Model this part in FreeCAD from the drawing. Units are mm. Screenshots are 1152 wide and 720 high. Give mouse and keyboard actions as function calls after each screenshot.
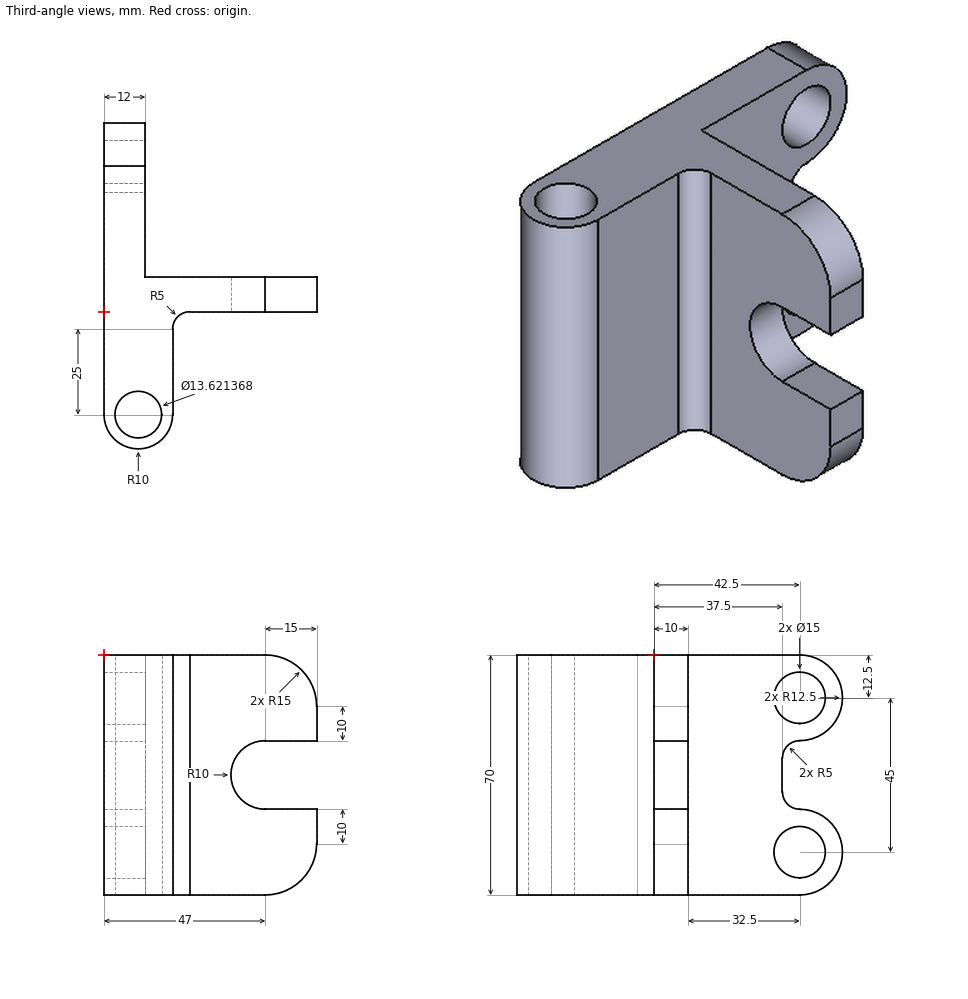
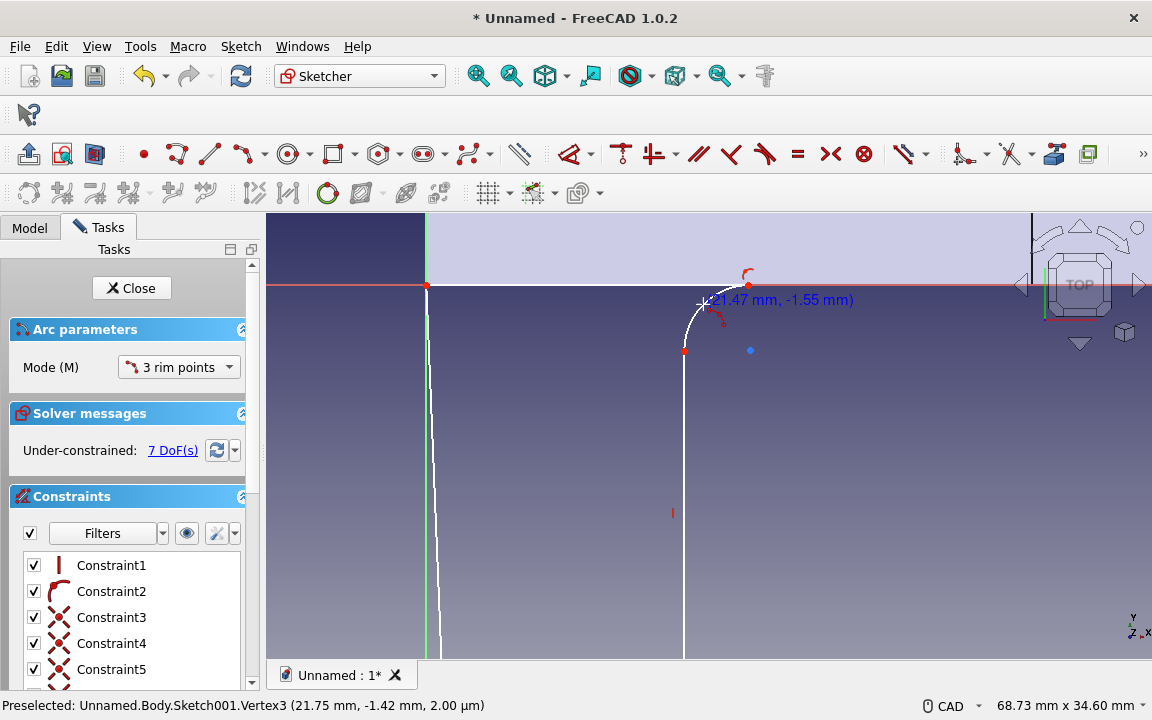
scroll(705, 306, down, 3)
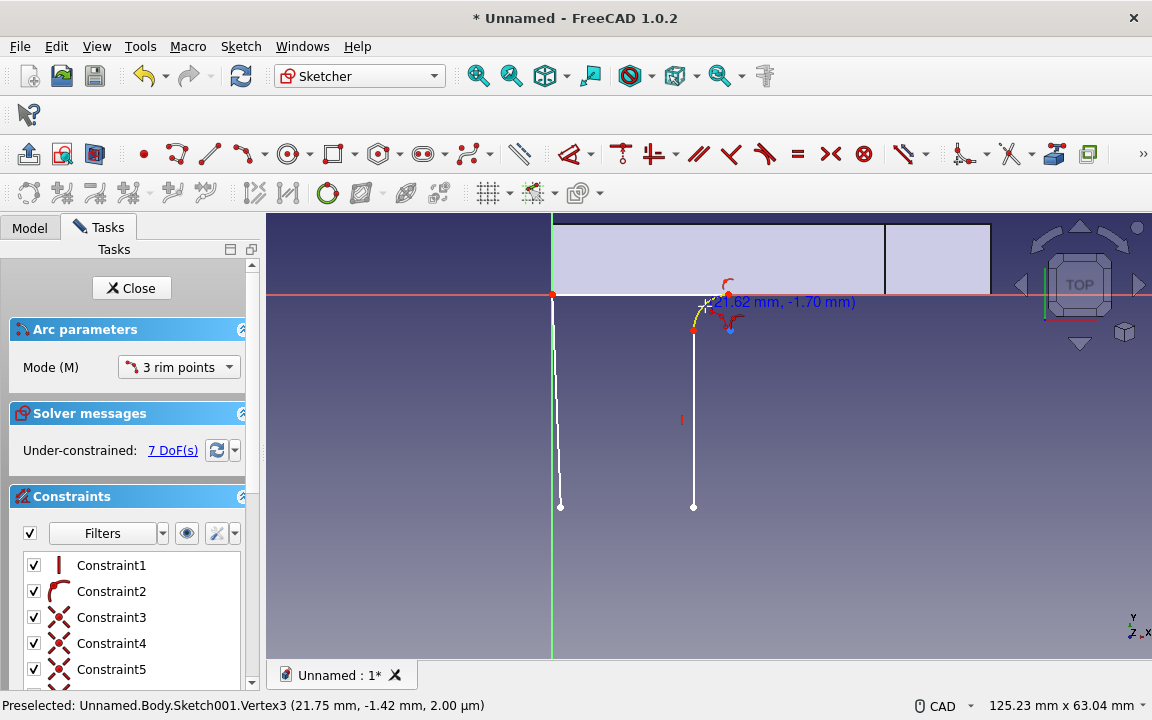
click(561, 508)
click(694, 508)
click(623, 578)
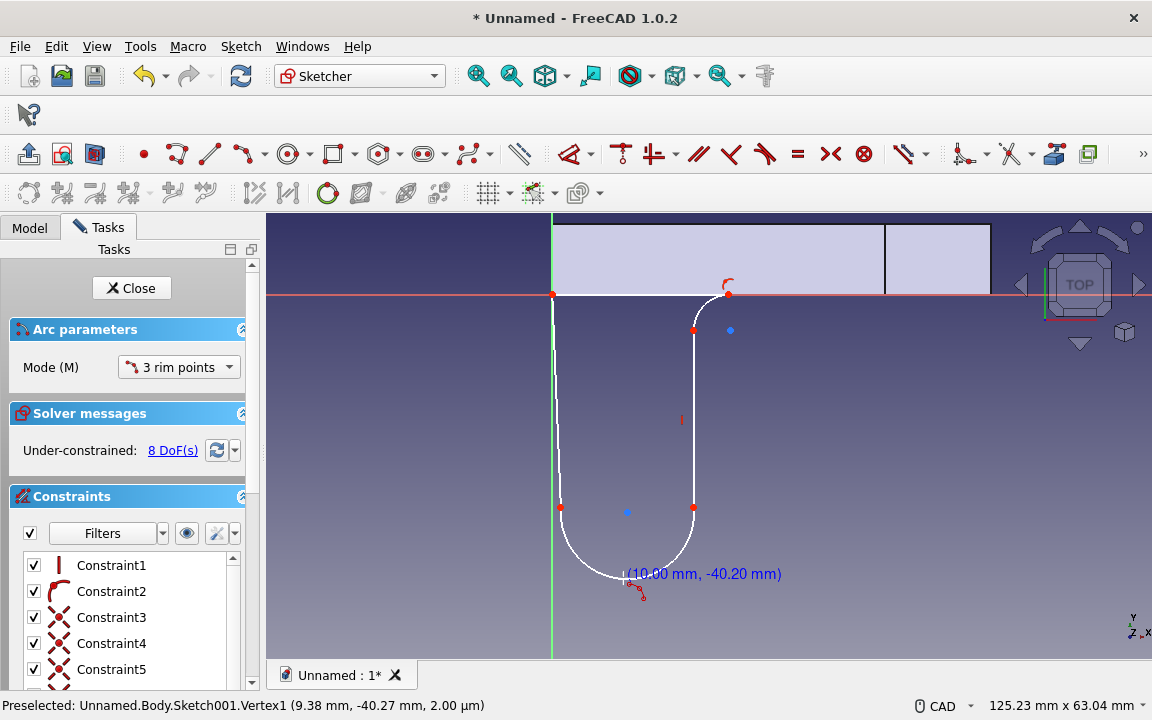
click(288, 154)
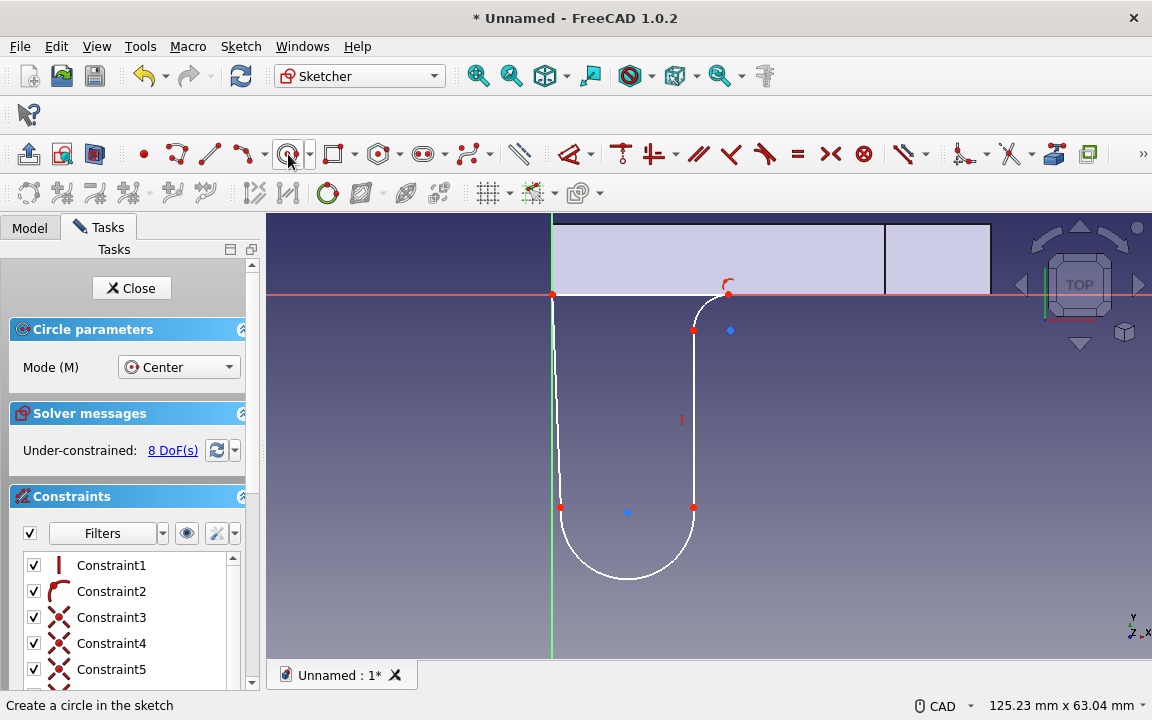
click(623, 507)
move(657, 473)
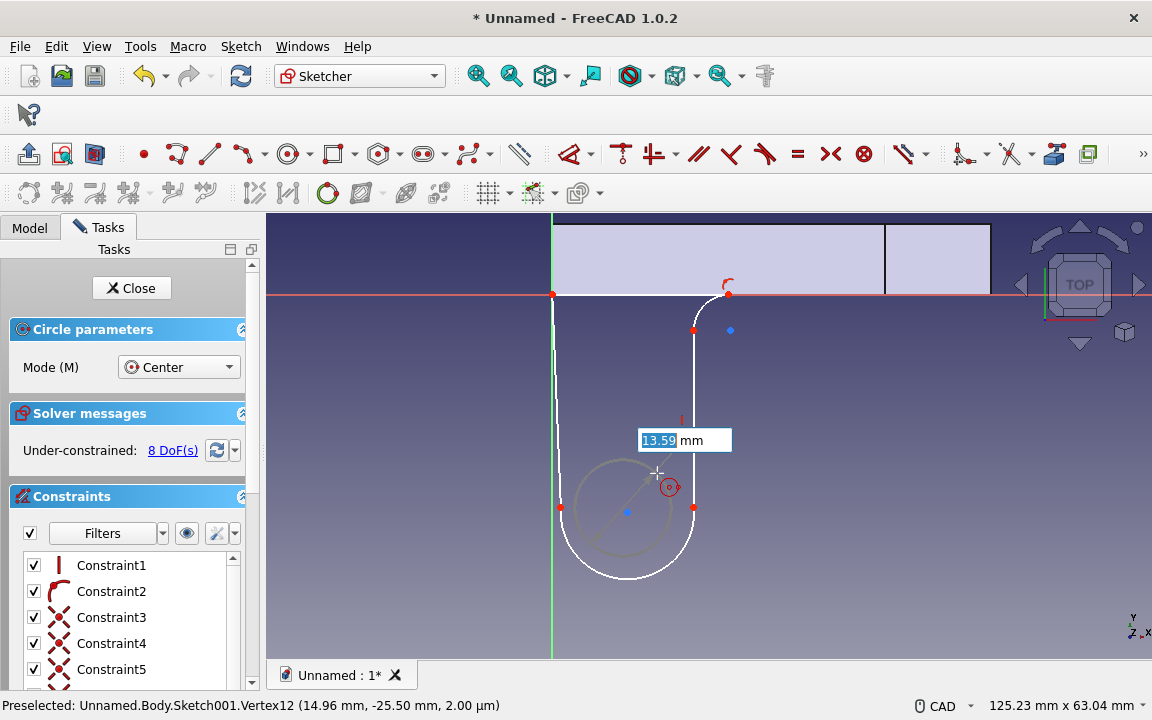
text(13.621368)
key(Return)
key(Escape)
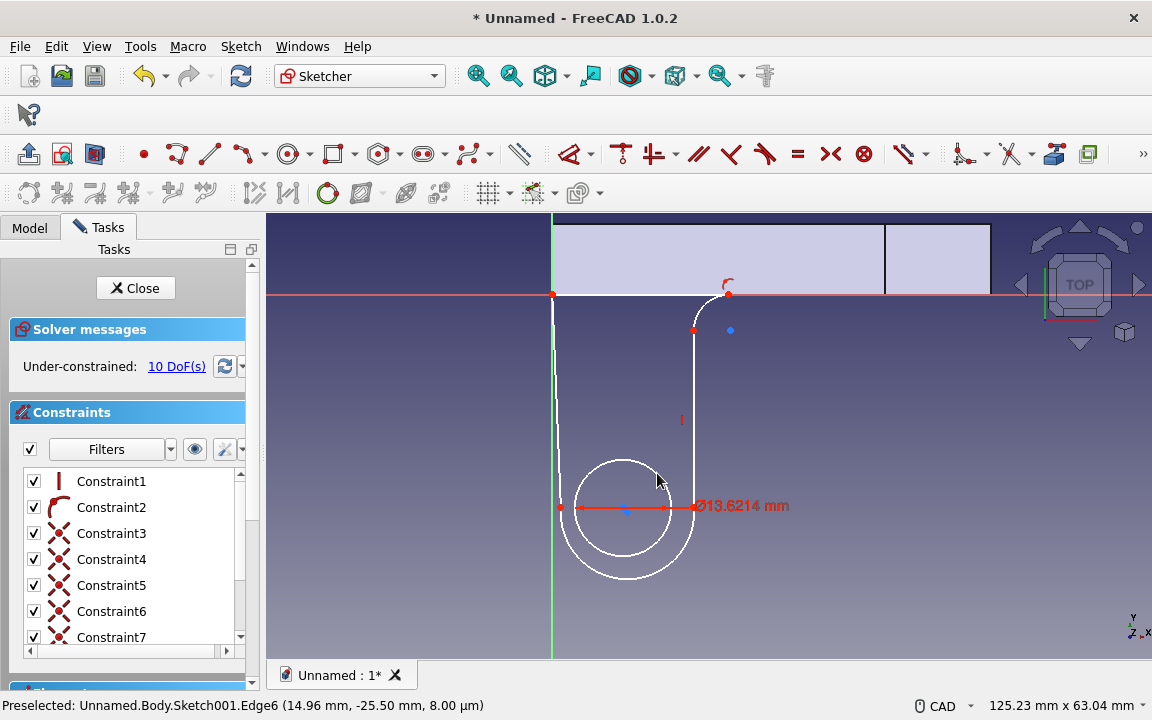
click(694, 455)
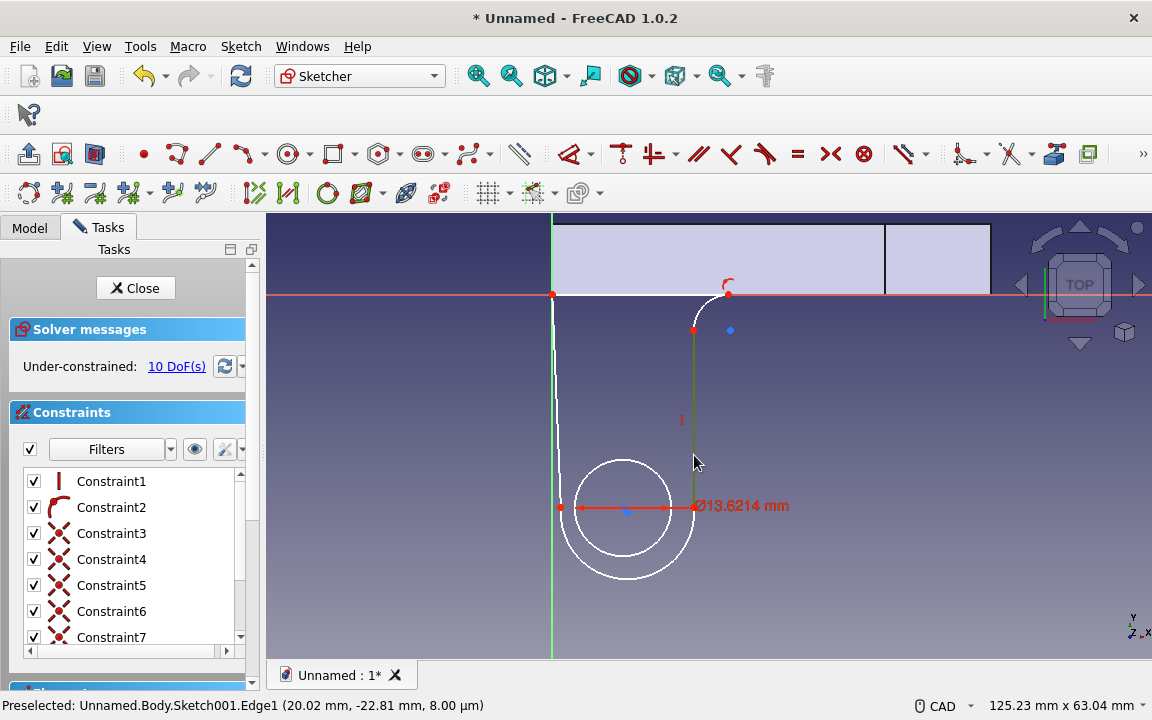
click(698, 315)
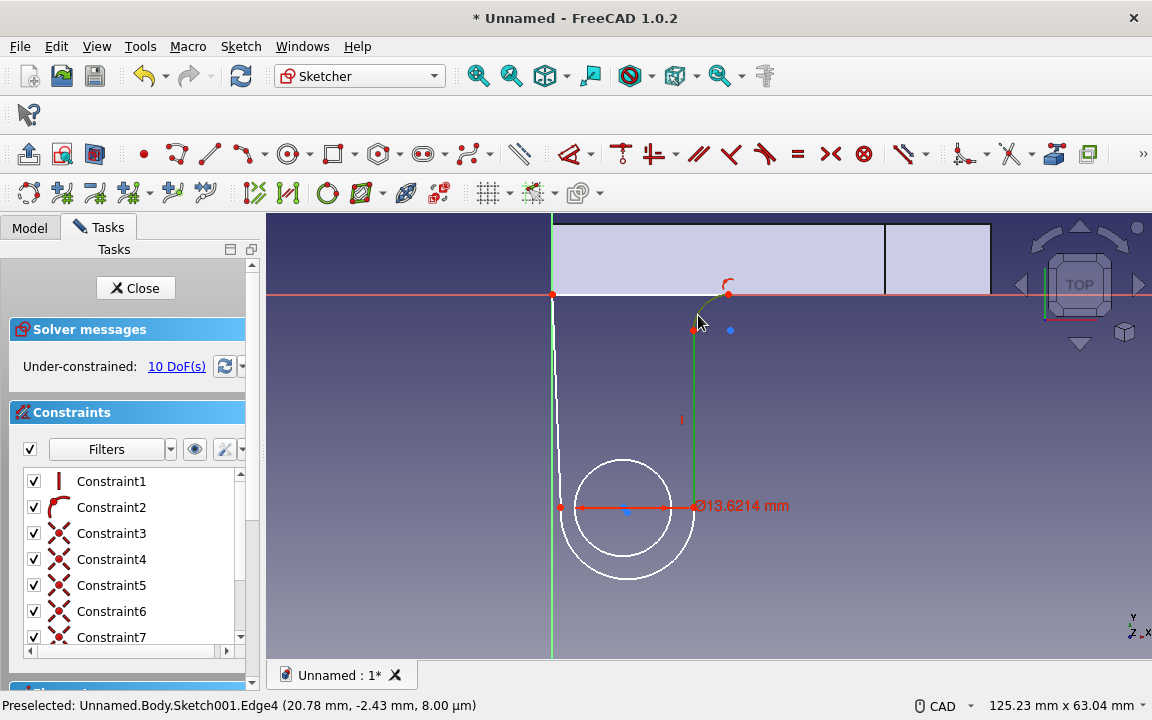
click(765, 154)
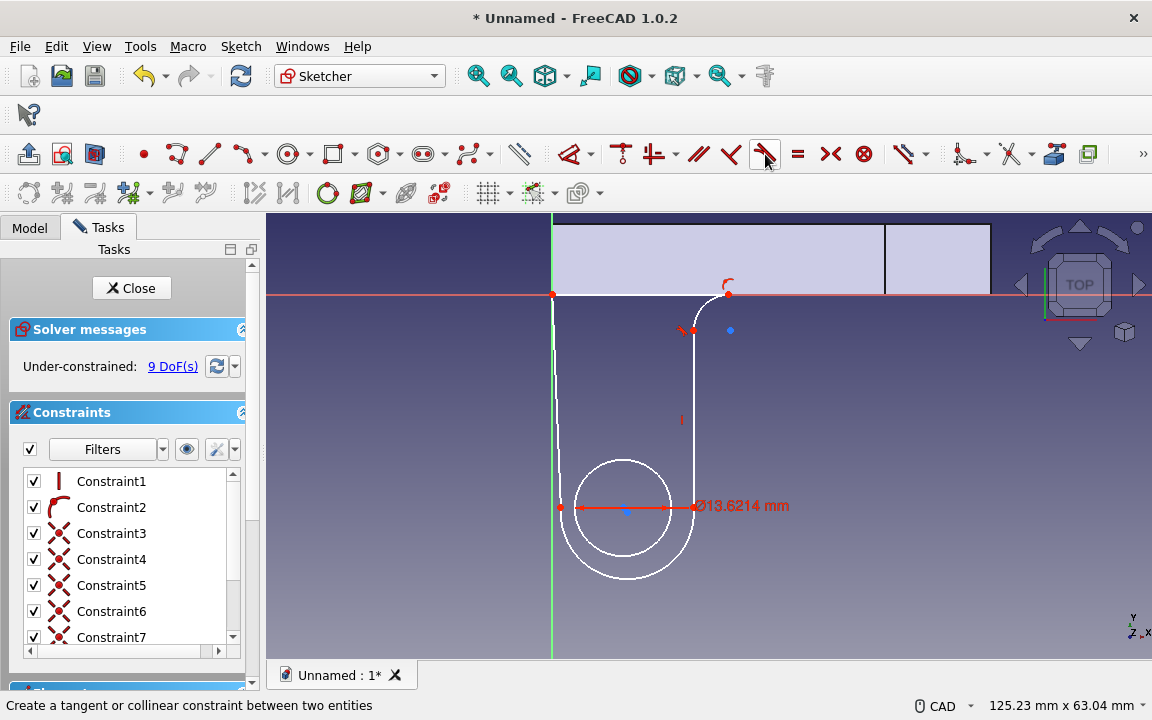
click(694, 455)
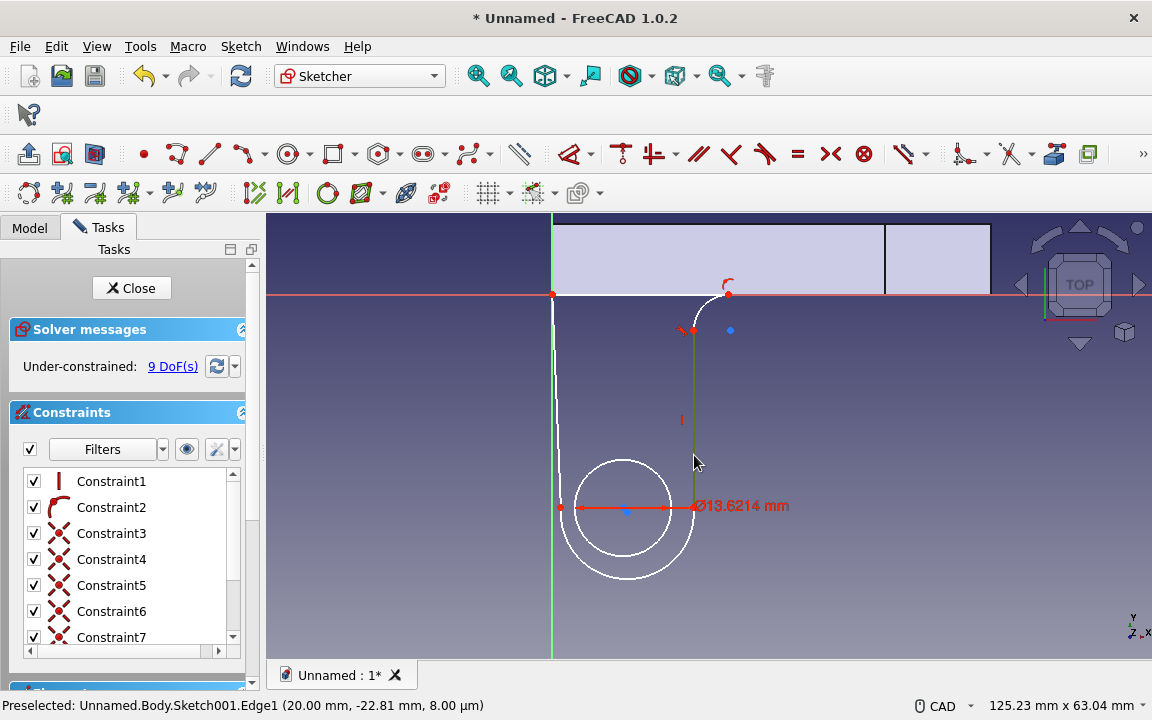
click(587, 565)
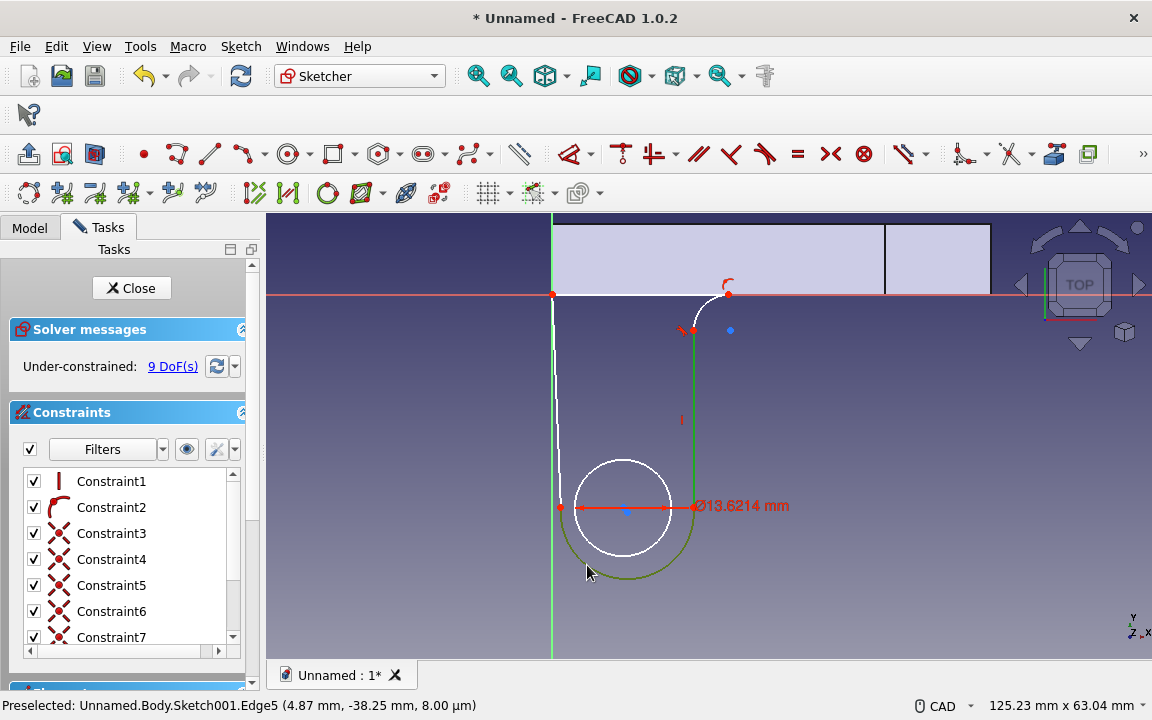
click(765, 154)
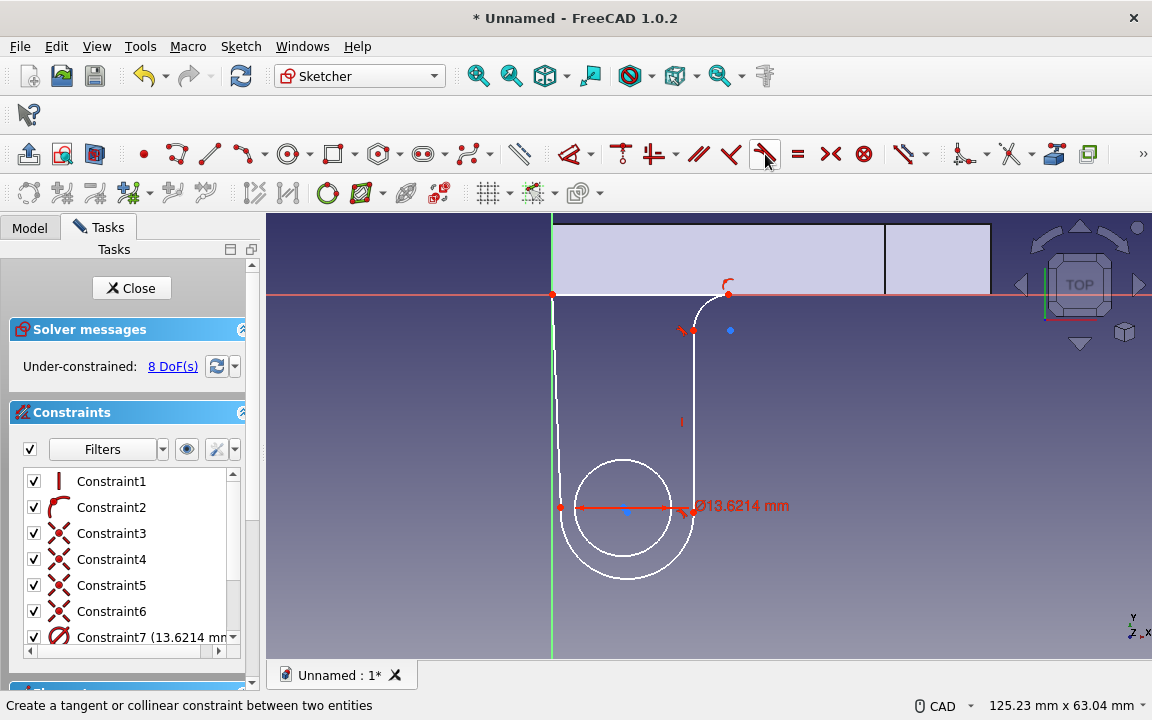
click(676, 295)